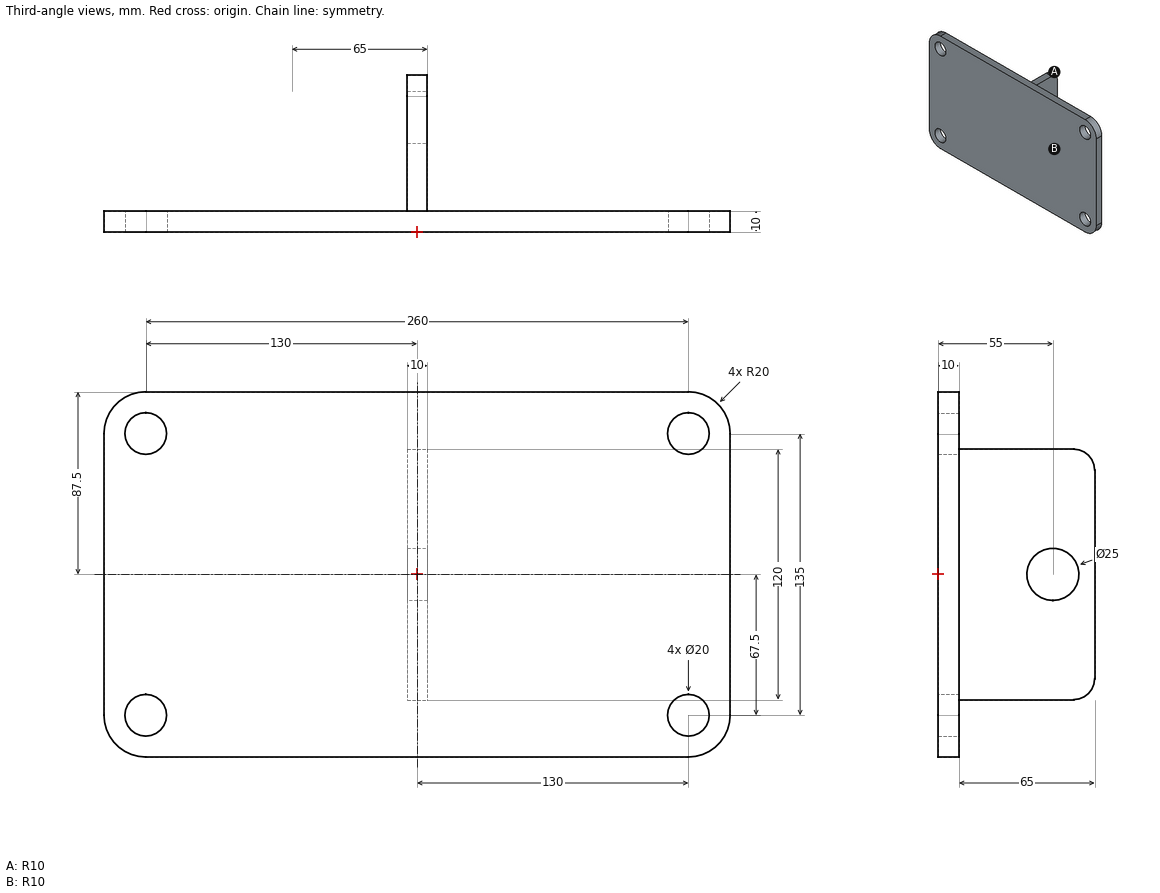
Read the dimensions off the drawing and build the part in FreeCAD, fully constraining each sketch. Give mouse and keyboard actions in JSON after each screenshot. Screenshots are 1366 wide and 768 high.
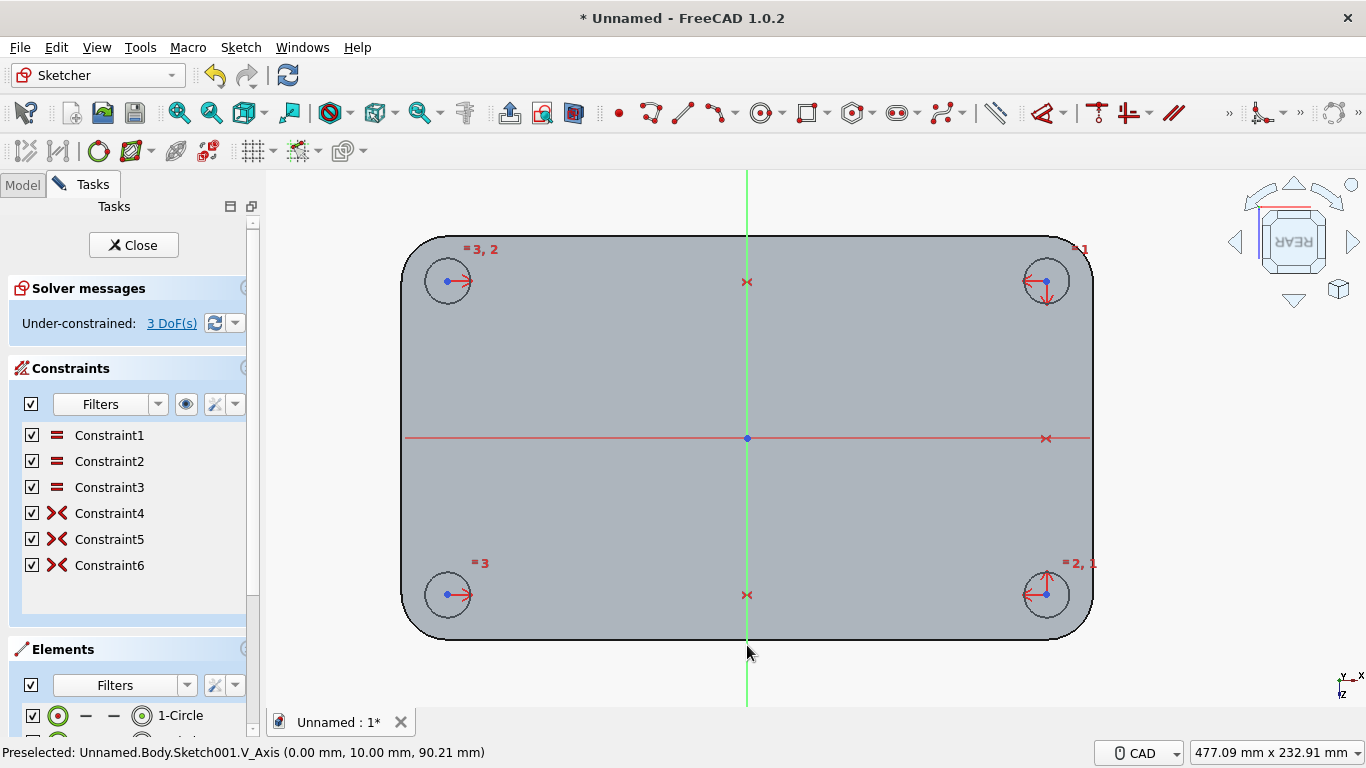
{"action": "left_click", "coordinate": [1042, 114]}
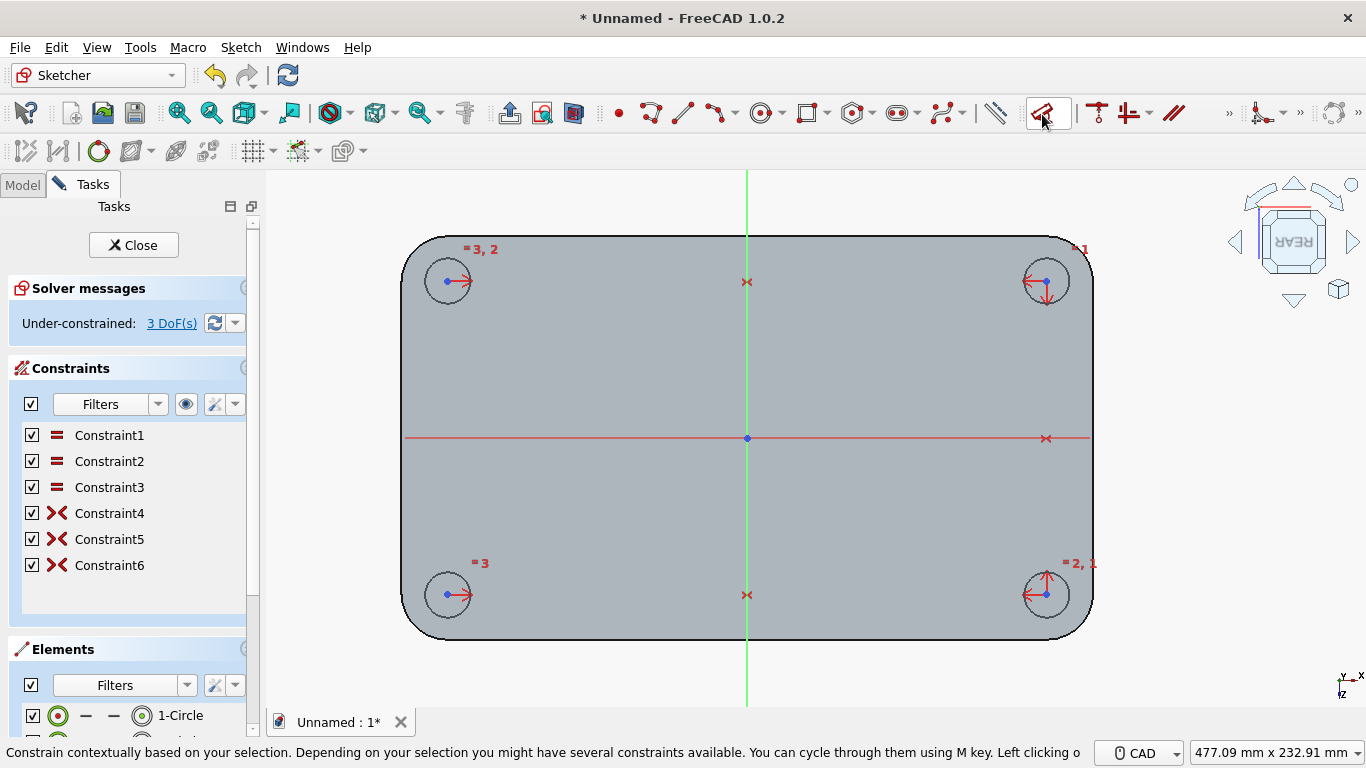
{"action": "left_click", "coordinate": [1063, 265]}
{"action": "left_click", "coordinate": [1086, 242]}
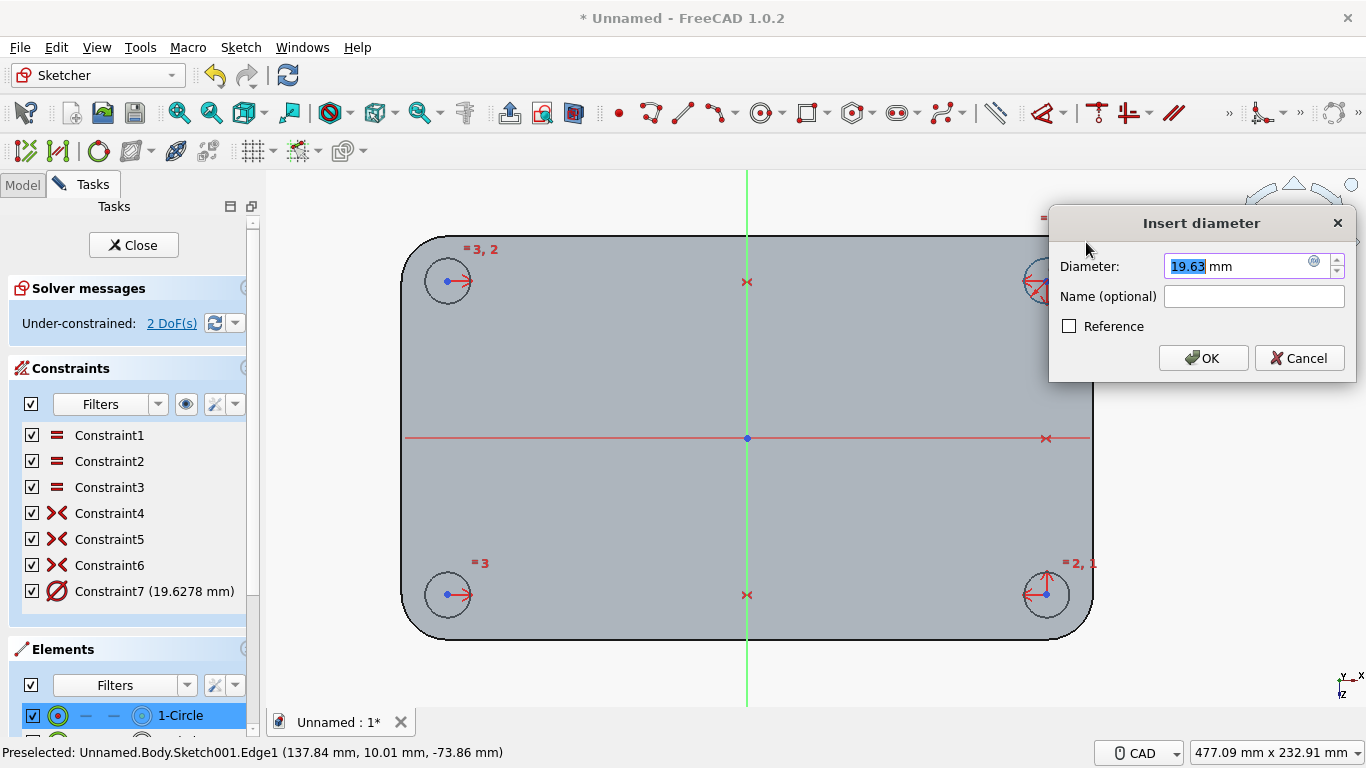
{"action": "type", "text": "20"}
{"action": "key", "text": "Return"}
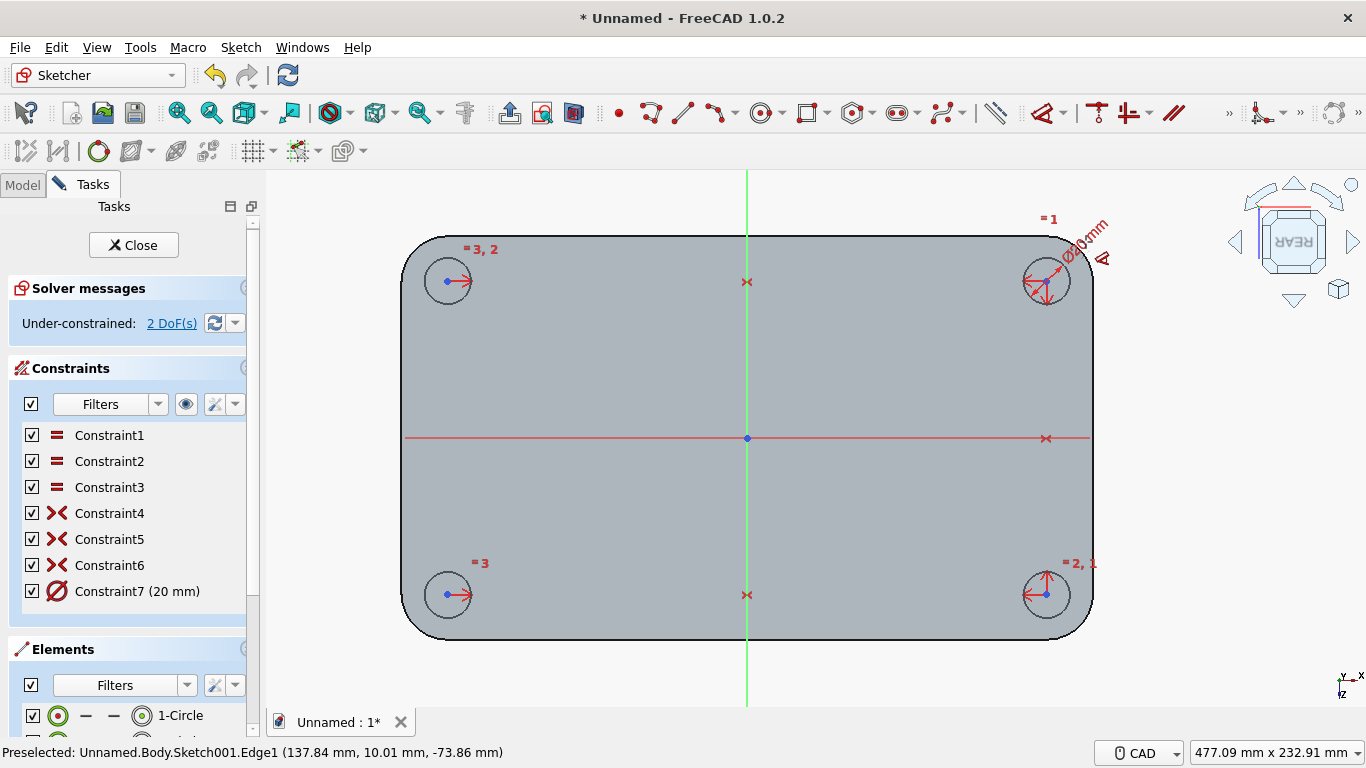
{"action": "left_click", "coordinate": [1047, 281]}
{"action": "left_click", "coordinate": [897, 247]}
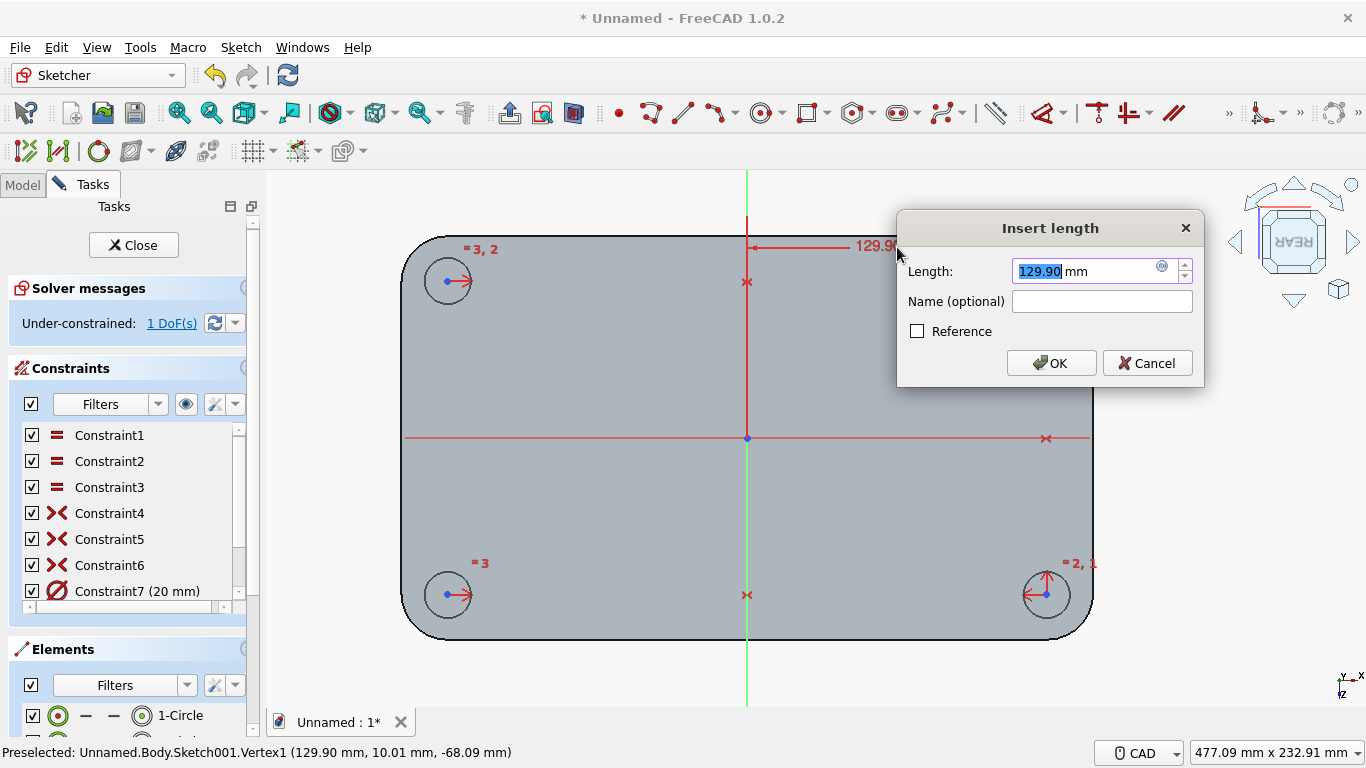
{"action": "type", "text": "130"}
{"action": "key", "text": "Return"}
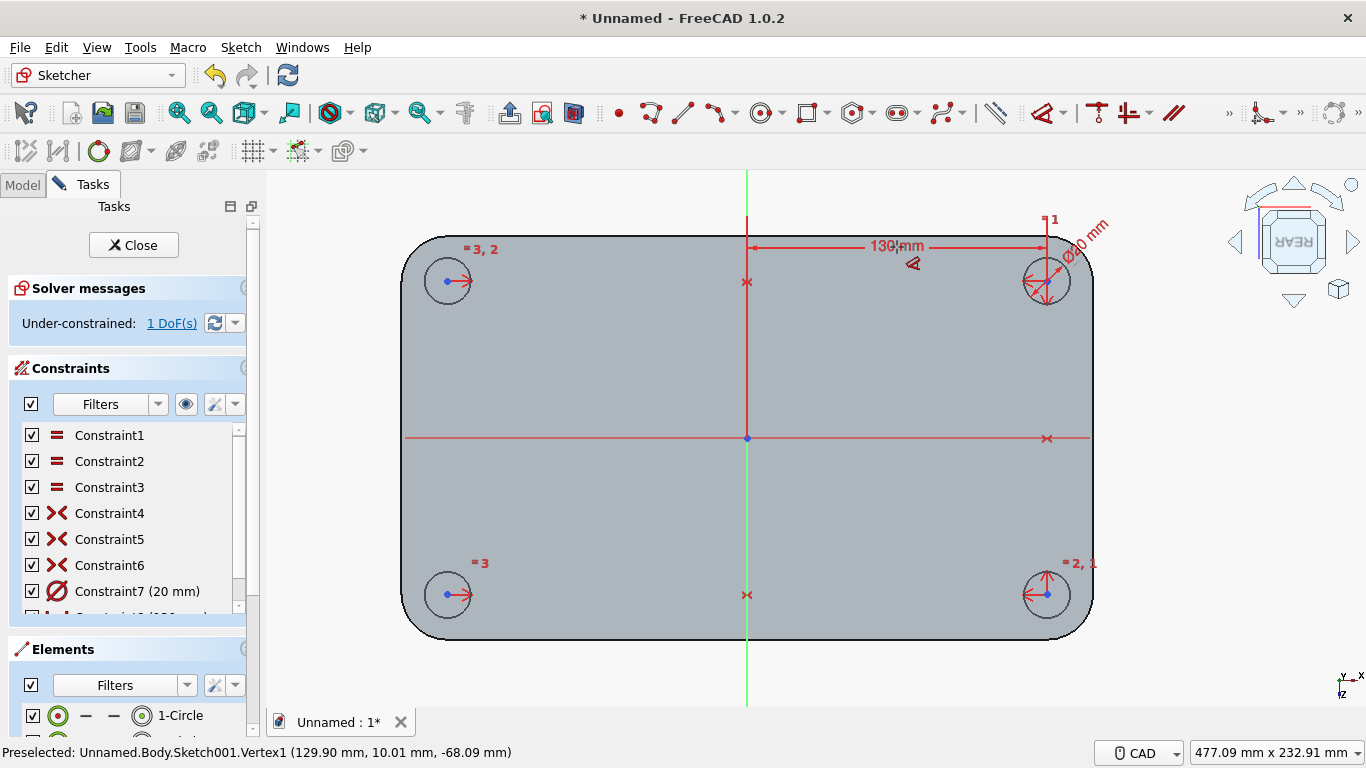
{"action": "left_click", "coordinate": [1047, 281]}
{"action": "left_click", "coordinate": [1081, 360]}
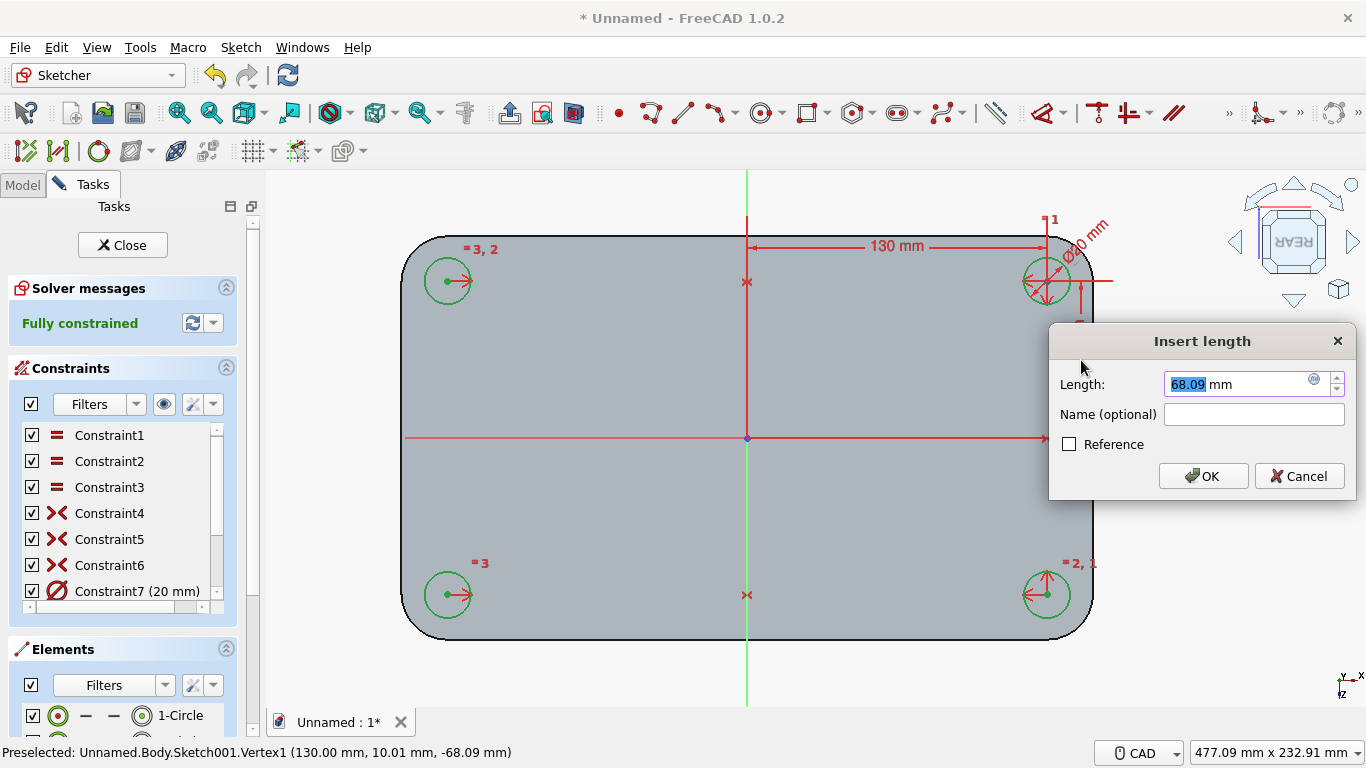
{"action": "type", "text": "67.5"}
{"action": "key", "text": "Return"}
{"action": "key", "text": "Escape"}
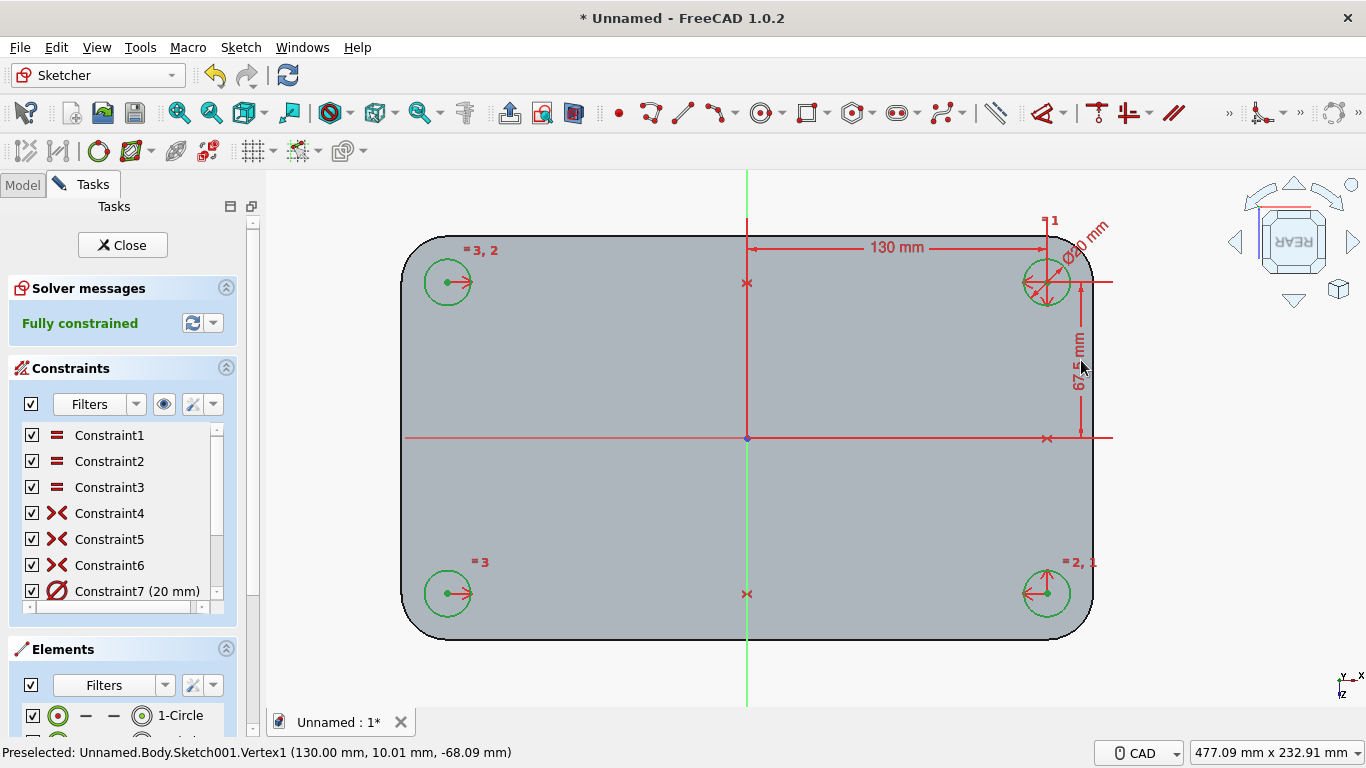
{"action": "left_click", "coordinate": [123, 245]}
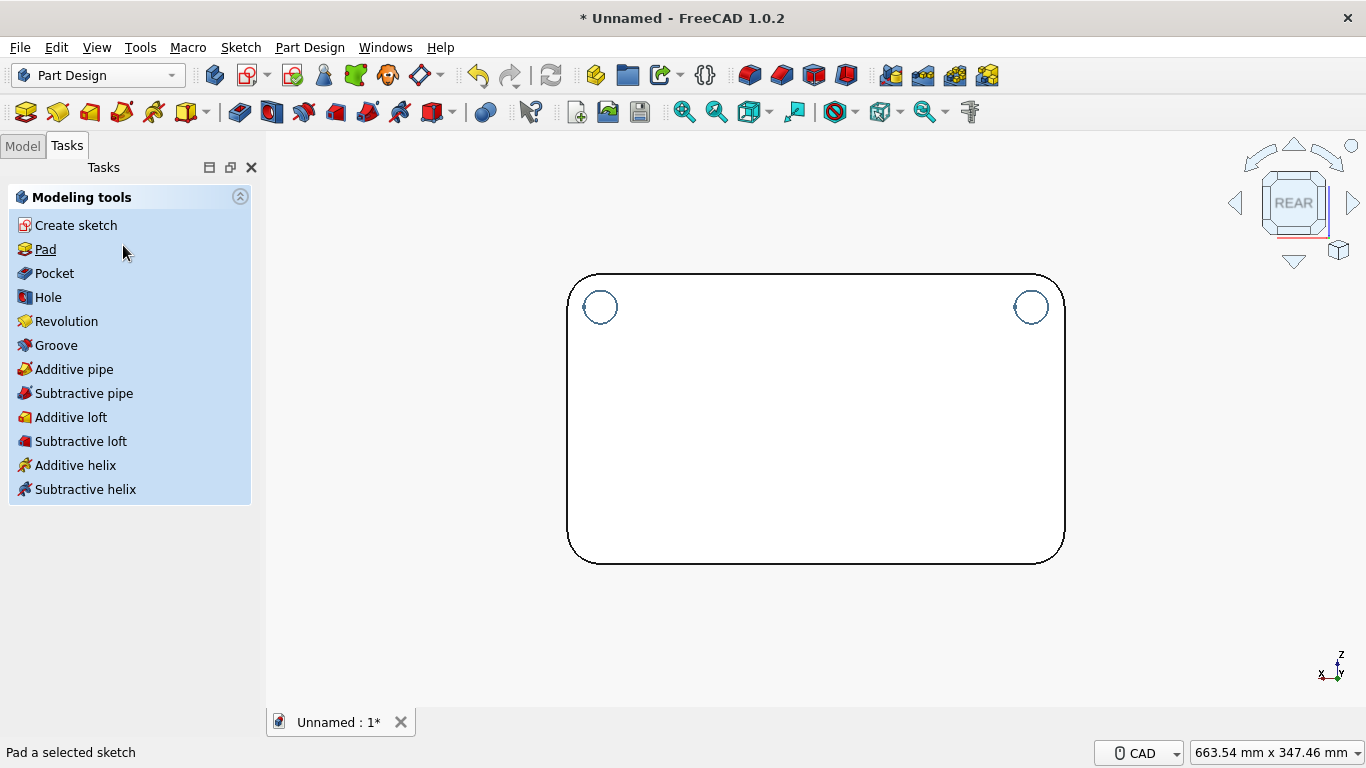
{"action": "left_click", "coordinate": [240, 112]}